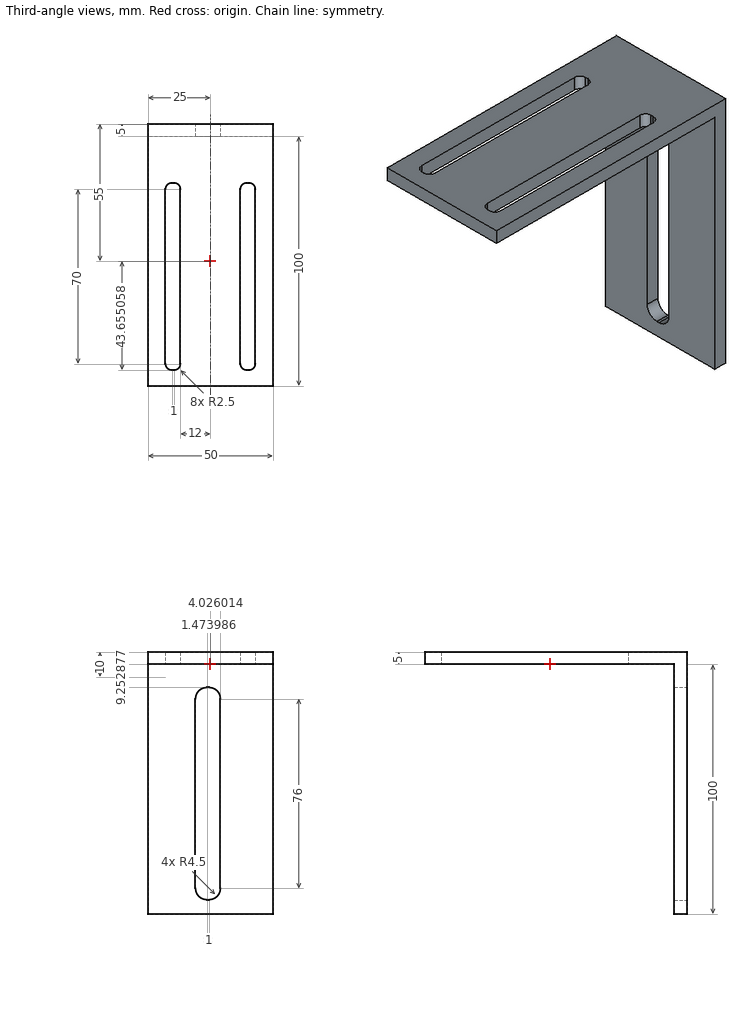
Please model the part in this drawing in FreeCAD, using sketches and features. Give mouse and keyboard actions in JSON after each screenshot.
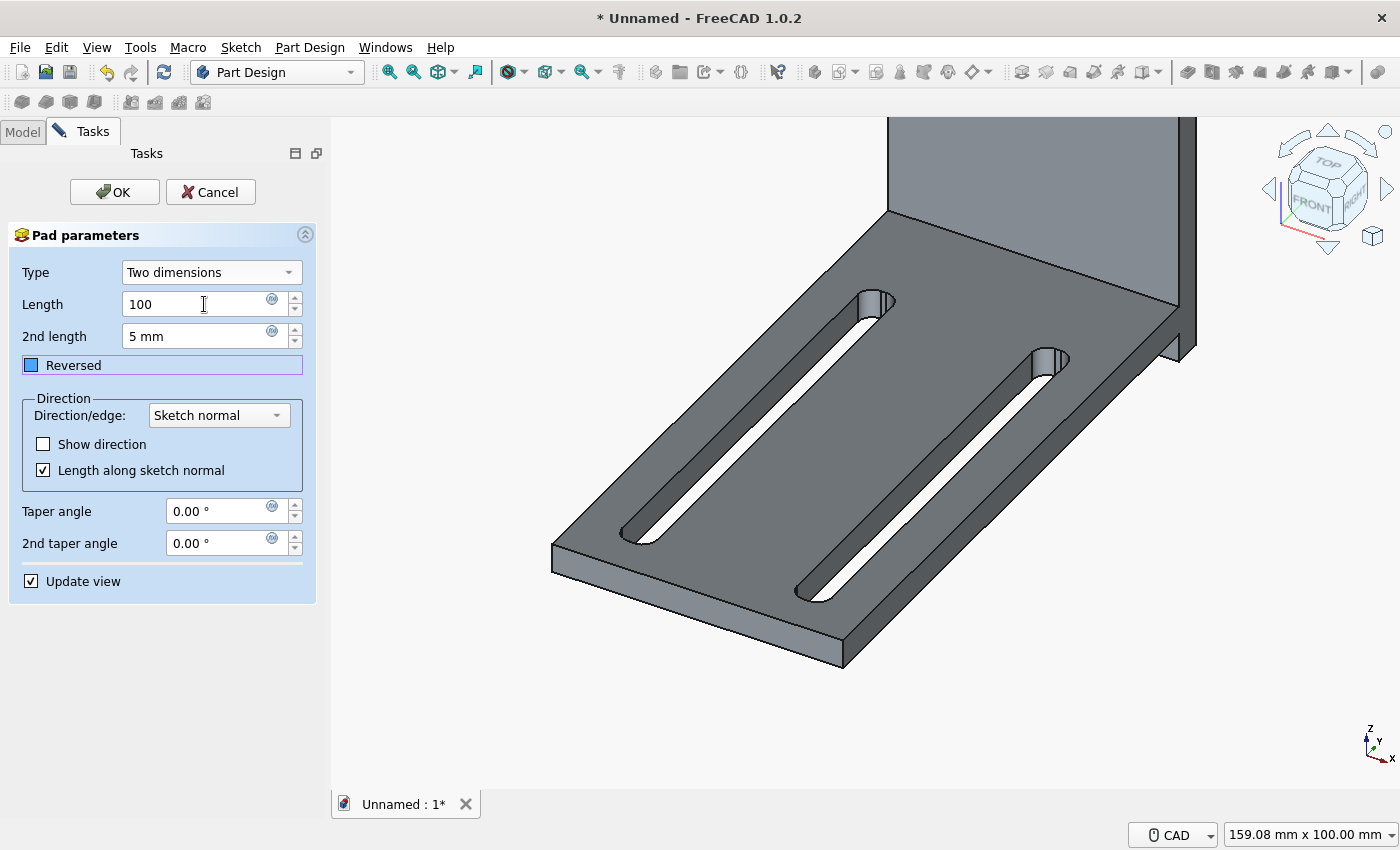
{"action": "left_click", "coordinate": [30, 365]}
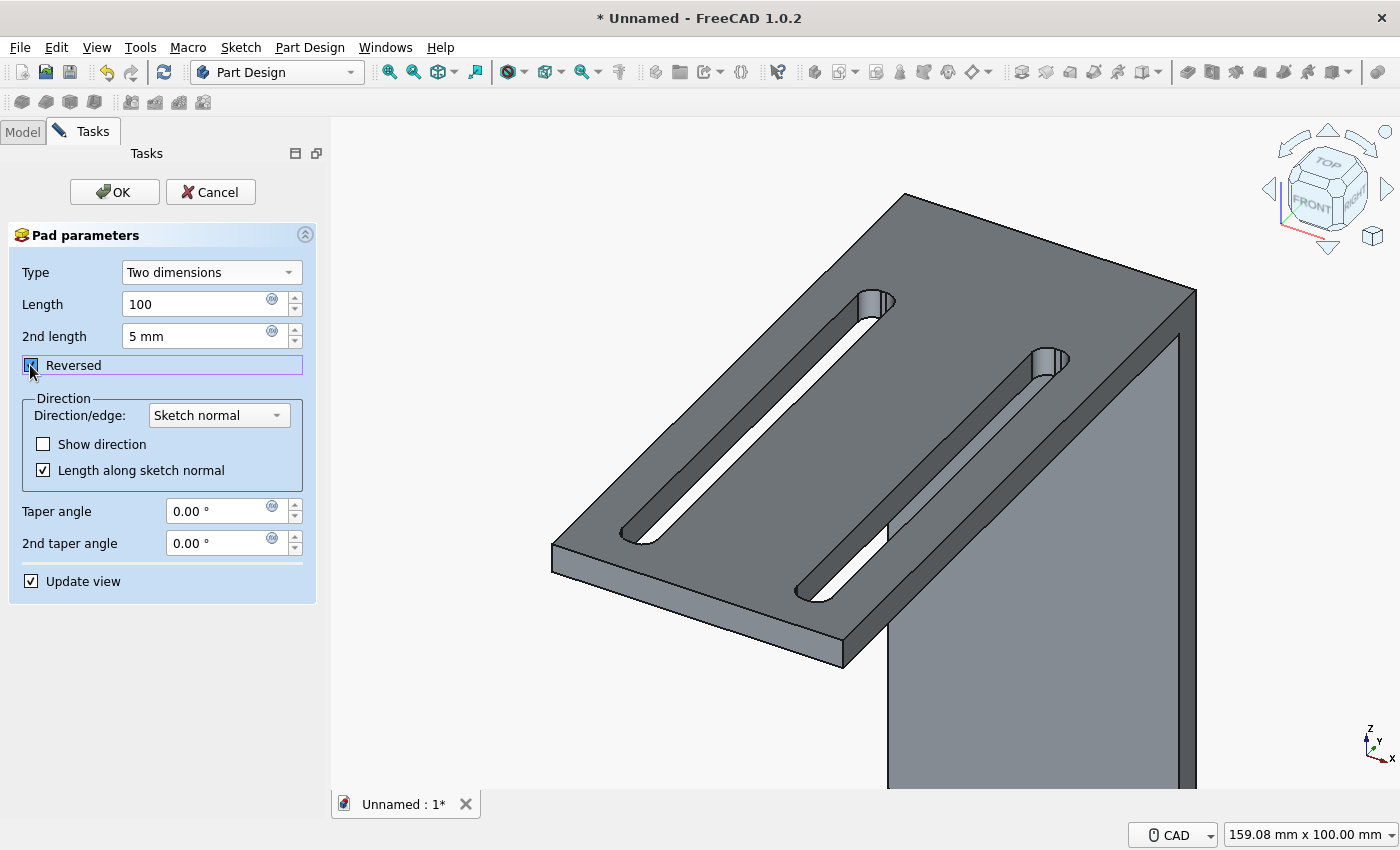
{"action": "left_click", "coordinate": [115, 192]}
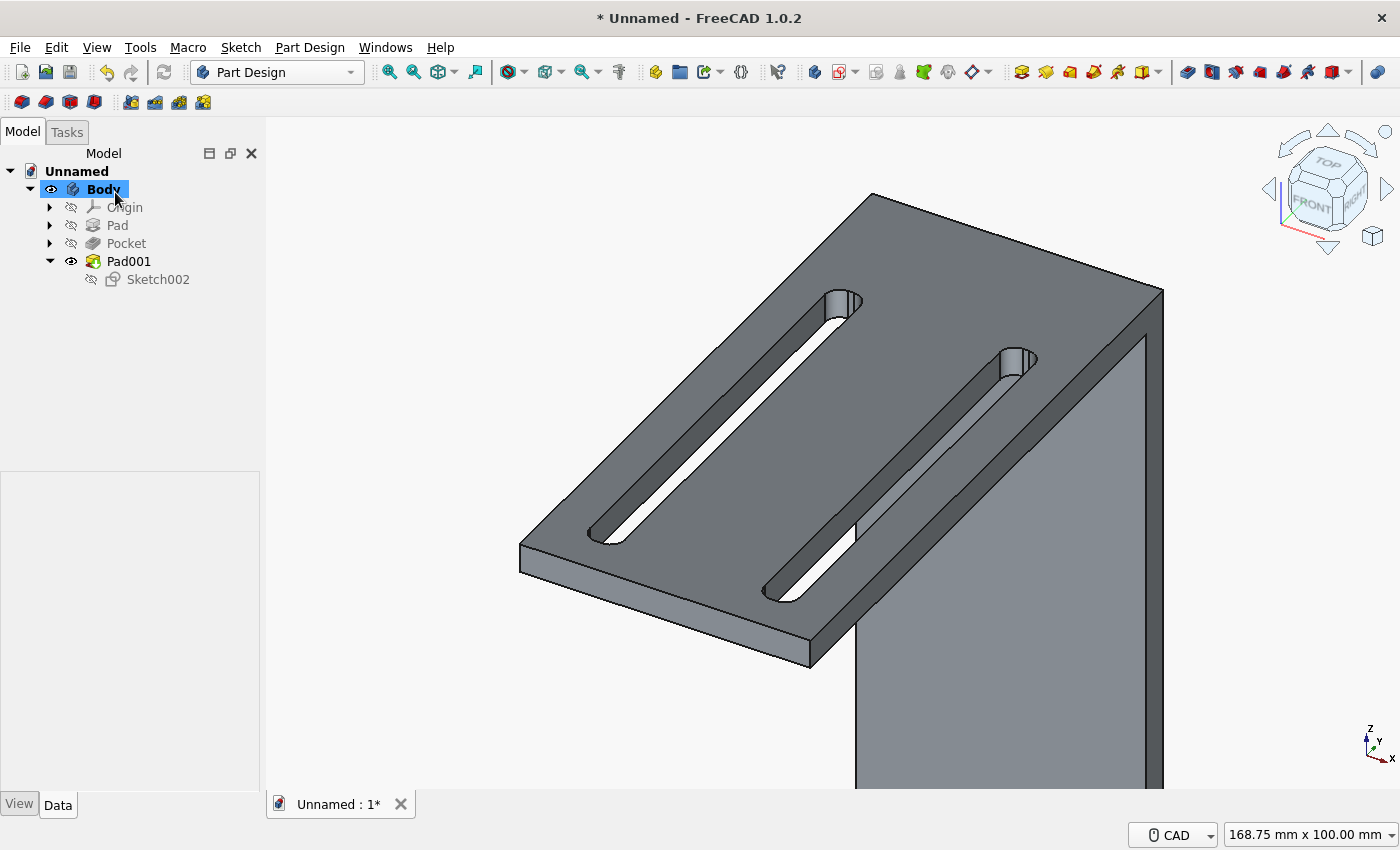
{"action": "key", "text": "v f"}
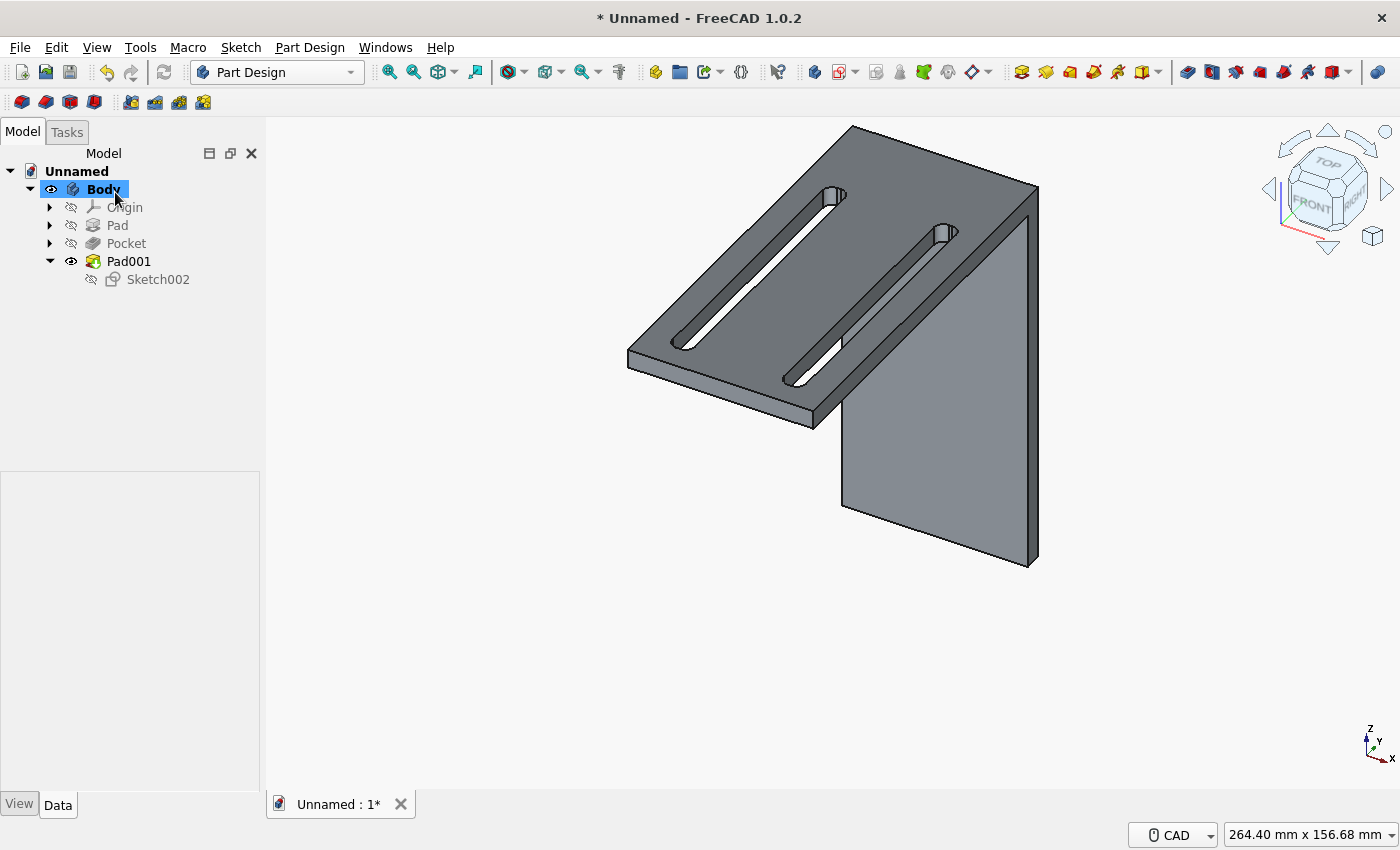
{"action": "left_click", "coordinate": [935, 360]}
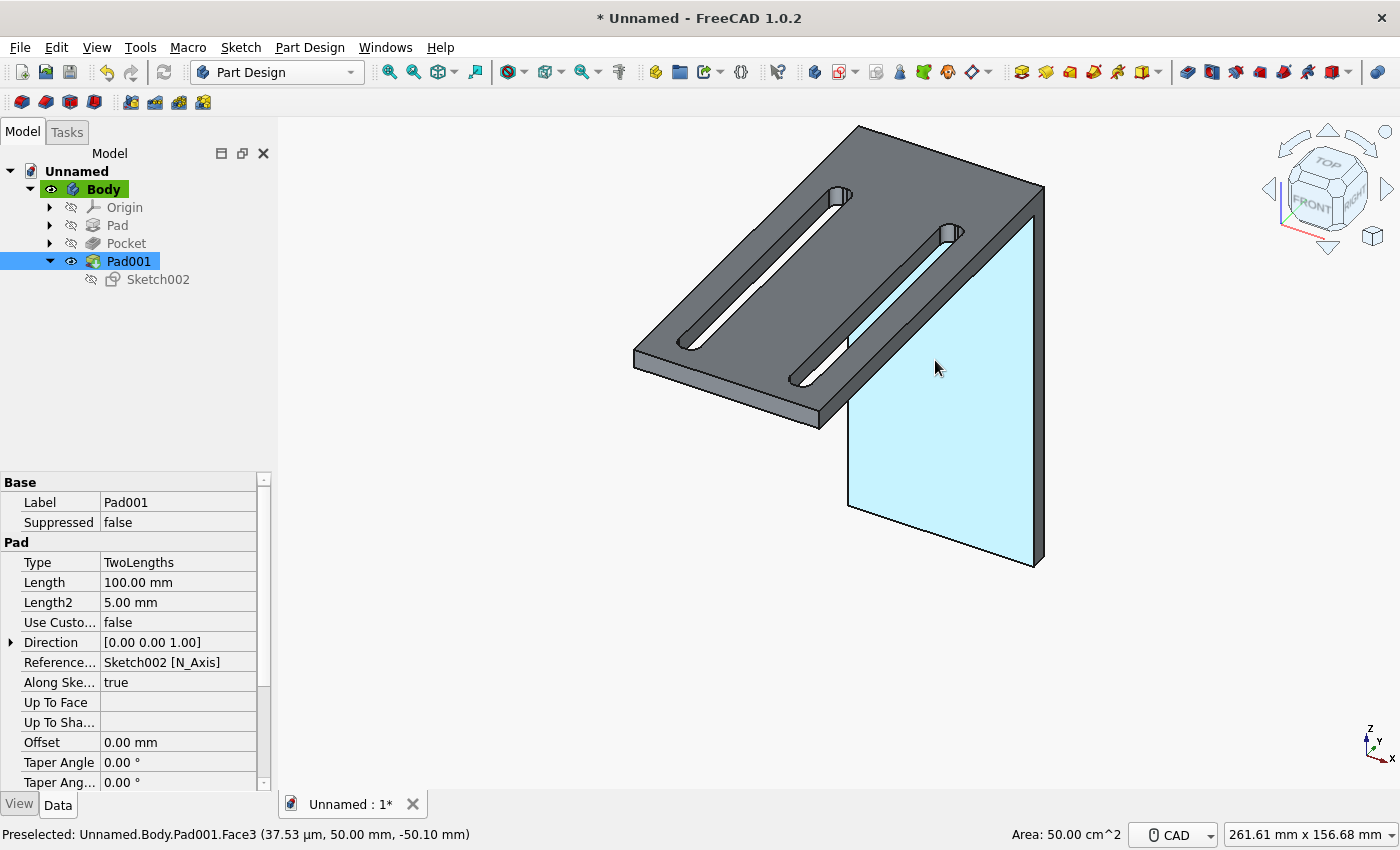
{"action": "left_click", "coordinate": [840, 72]}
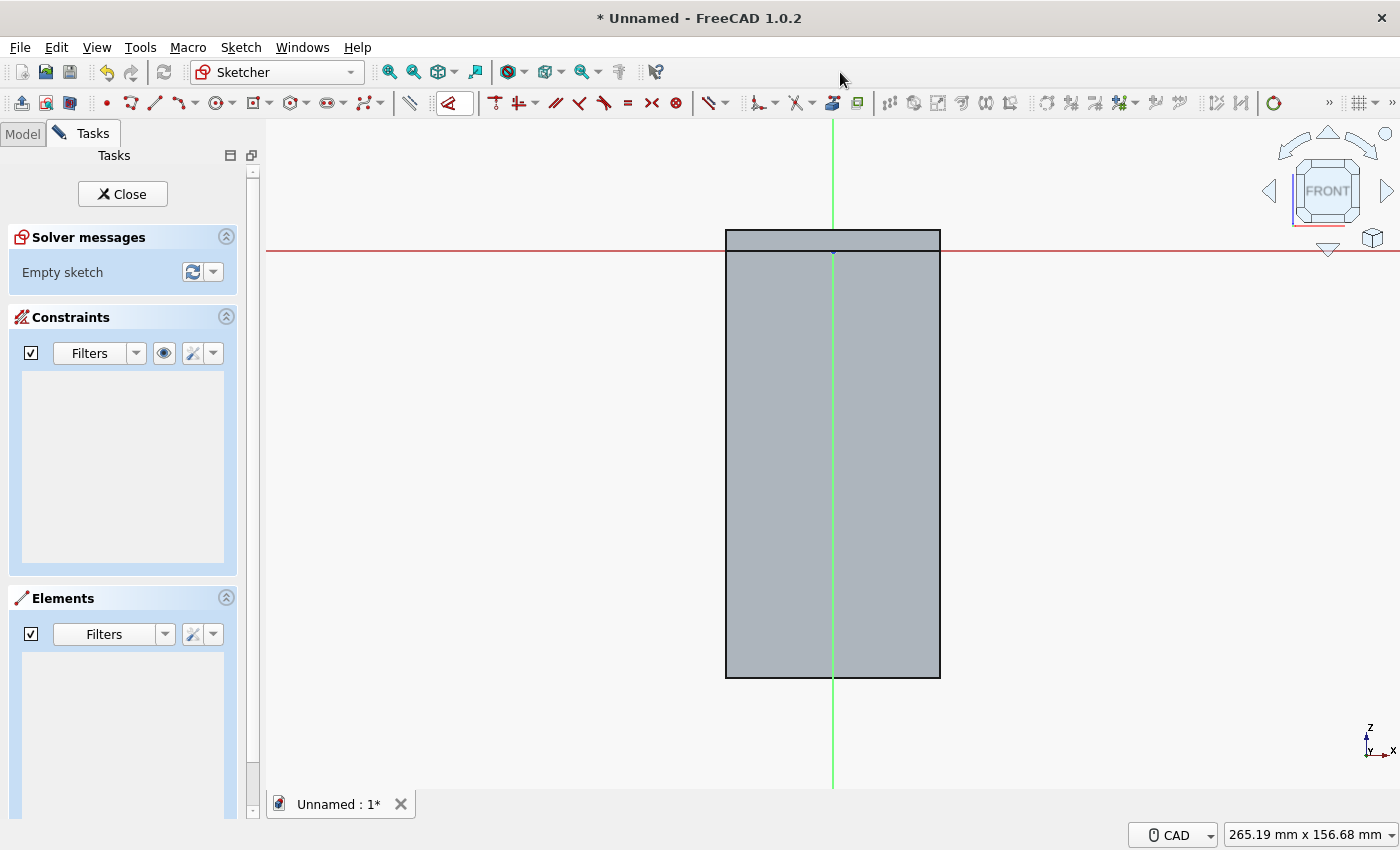
{"action": "left_click", "coordinate": [70, 104]}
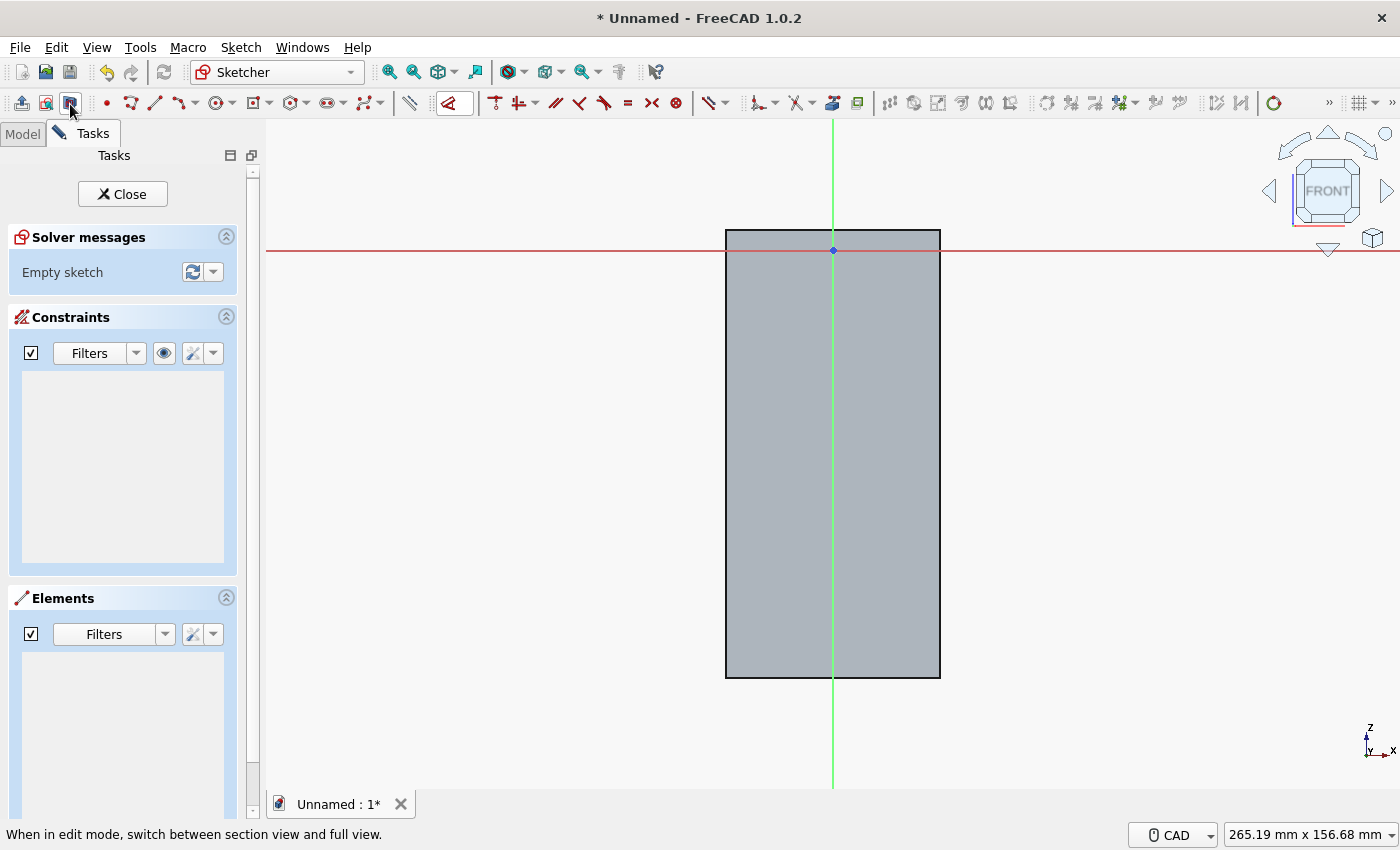
{"action": "key", "text": "g l"}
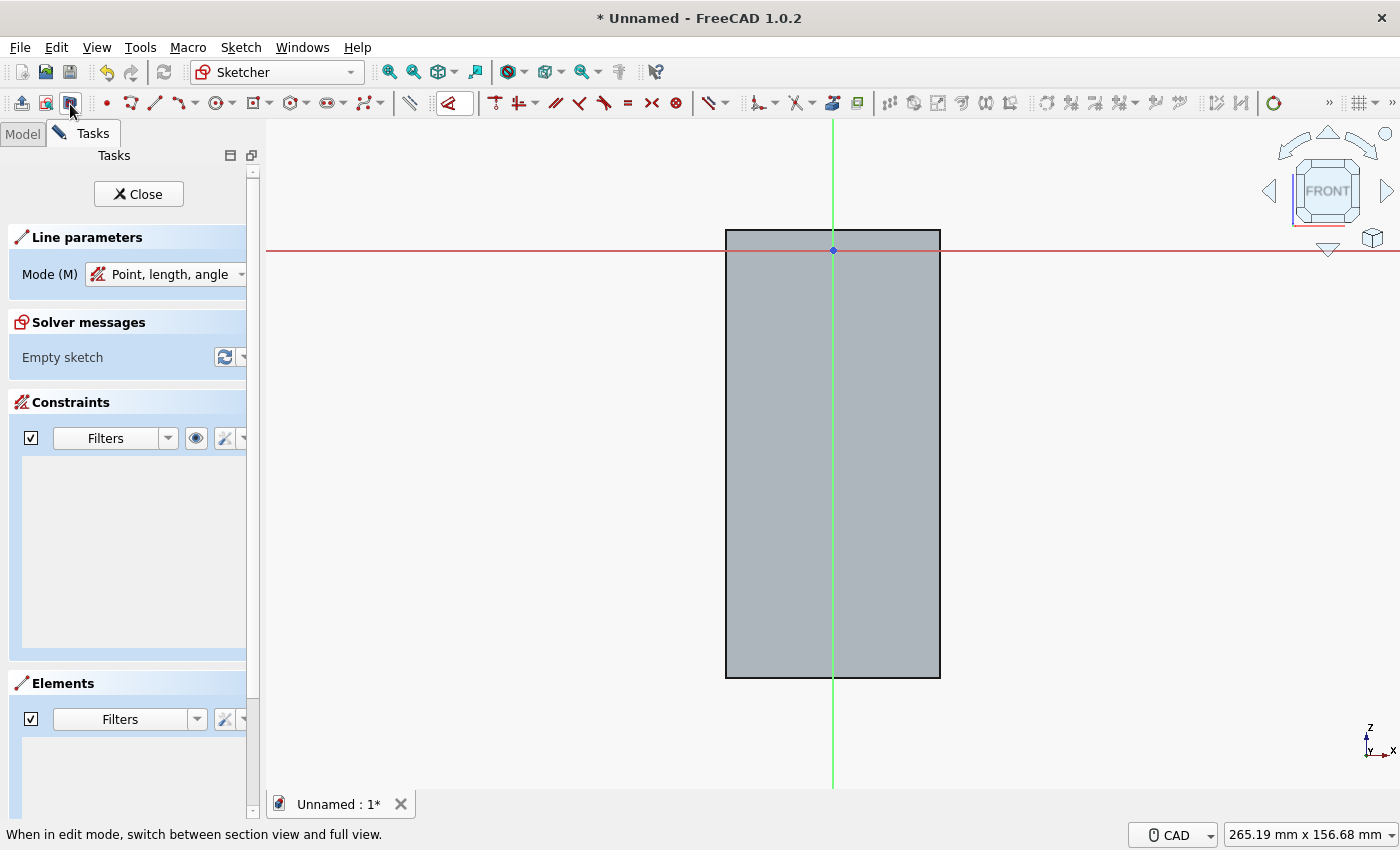
{"action": "scroll", "coordinate": [827, 654], "scroll_direction": "up", "scroll_amount": 5}